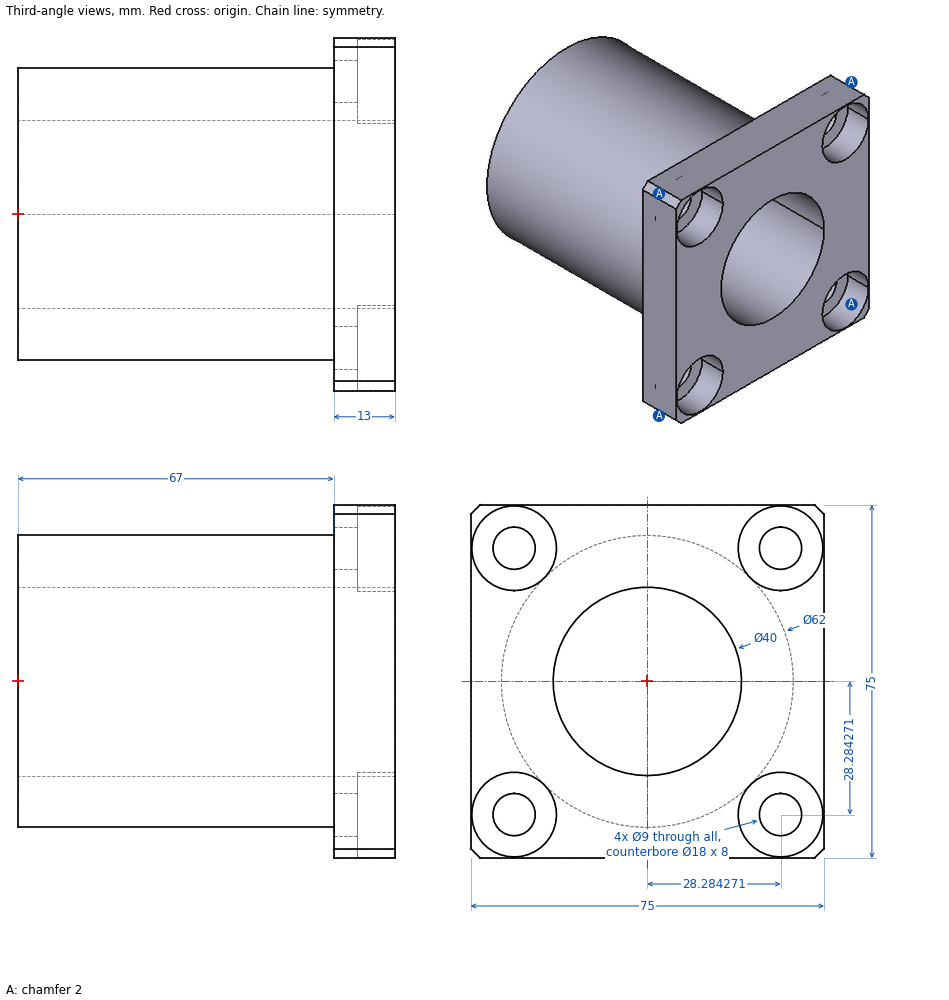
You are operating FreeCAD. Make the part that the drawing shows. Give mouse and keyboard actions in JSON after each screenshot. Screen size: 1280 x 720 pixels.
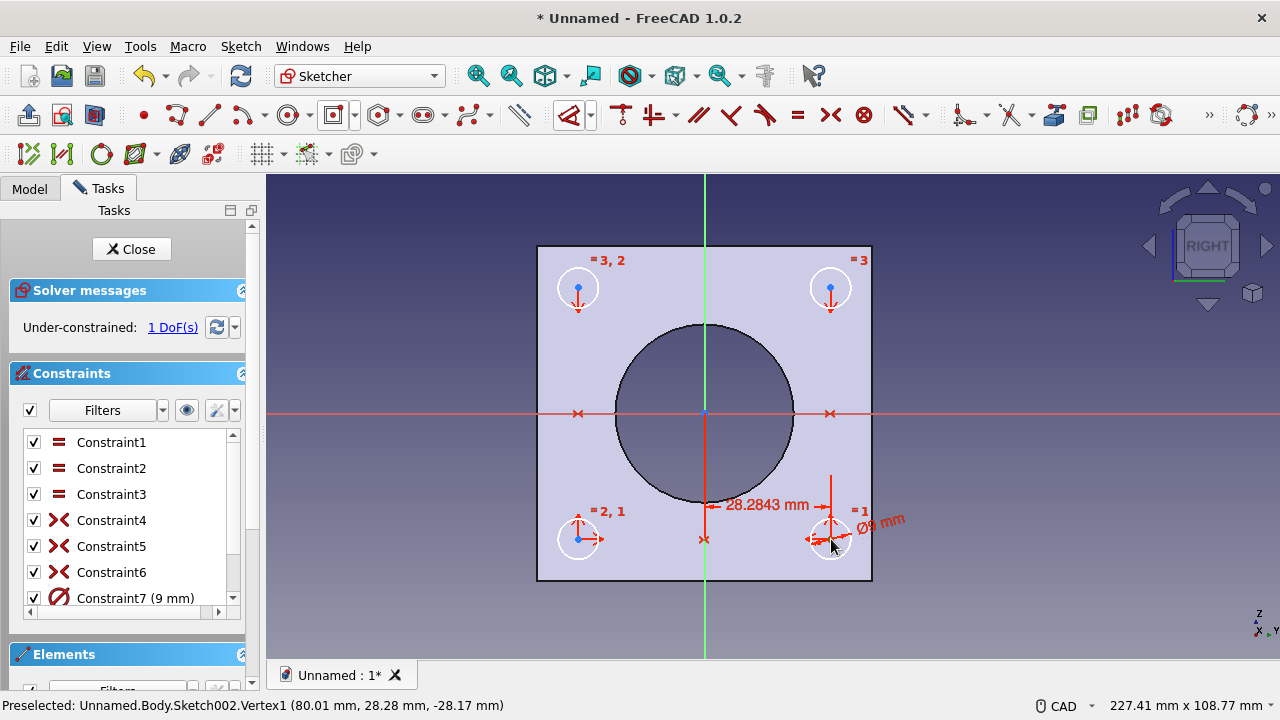
{"action": "key", "text": "i"}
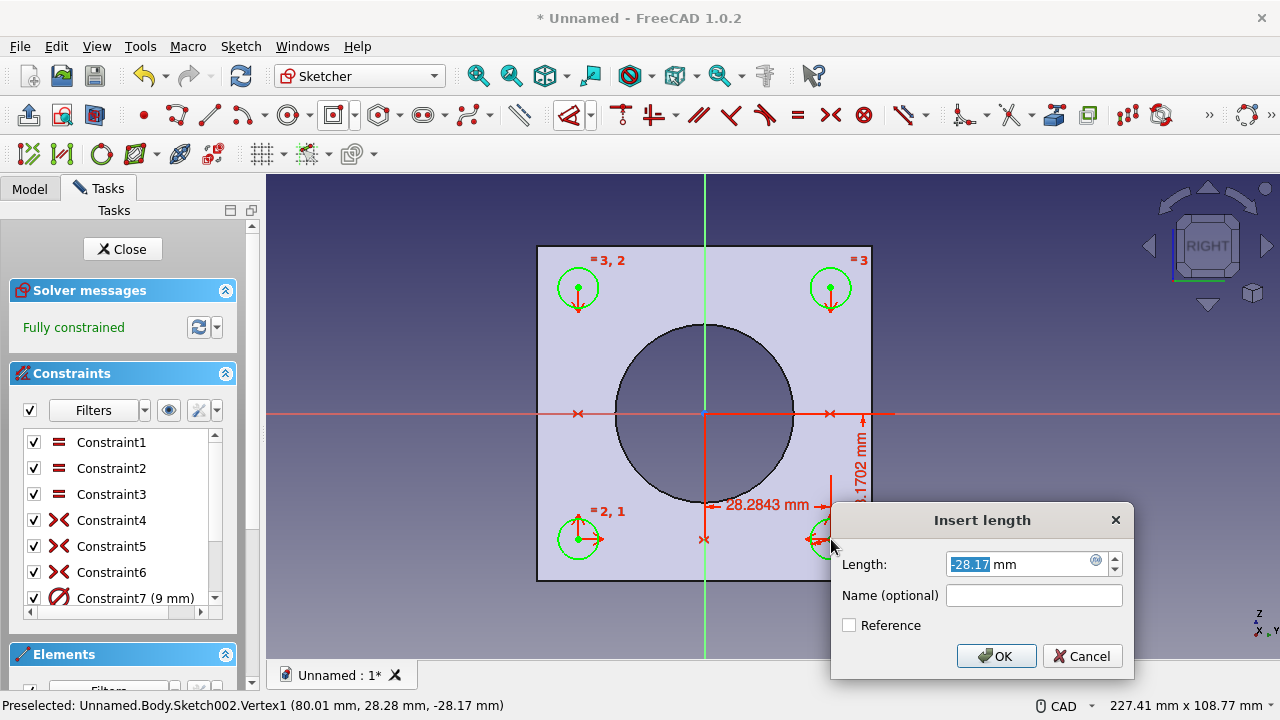
{"action": "type", "text": "-28.284271"}
{"action": "key", "text": "Return"}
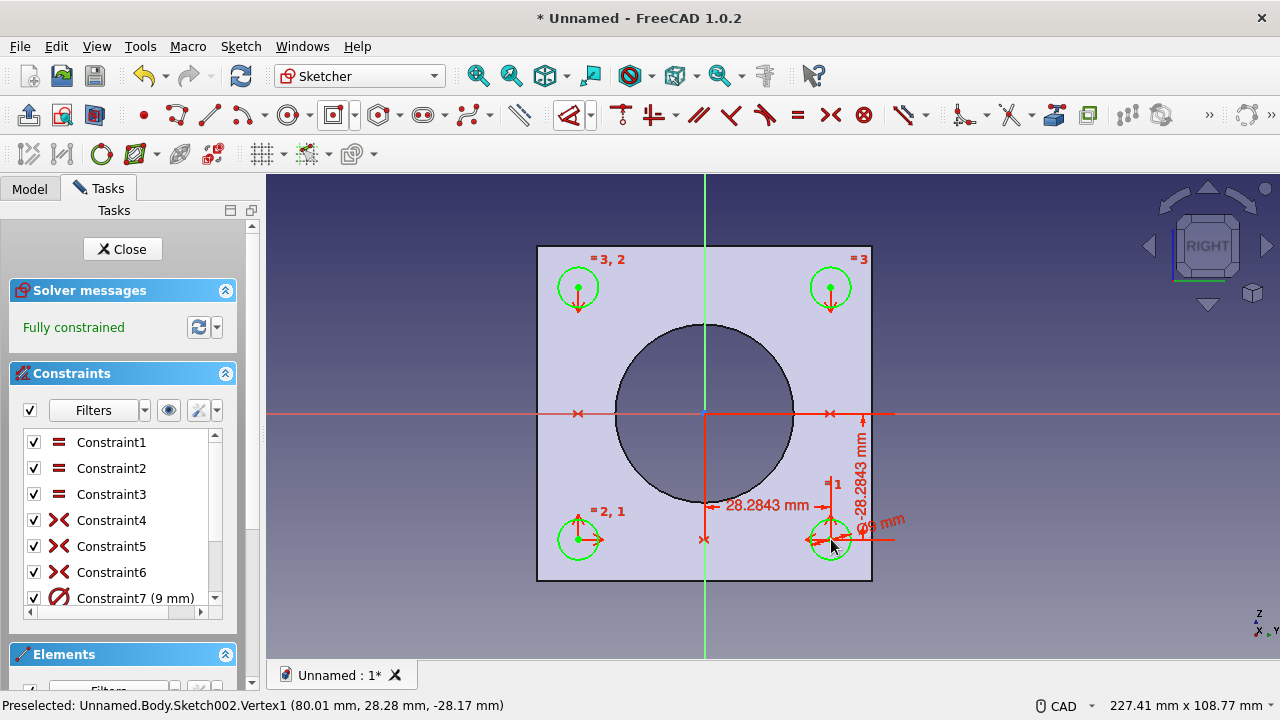
{"action": "left_click", "coordinate": [123, 249]}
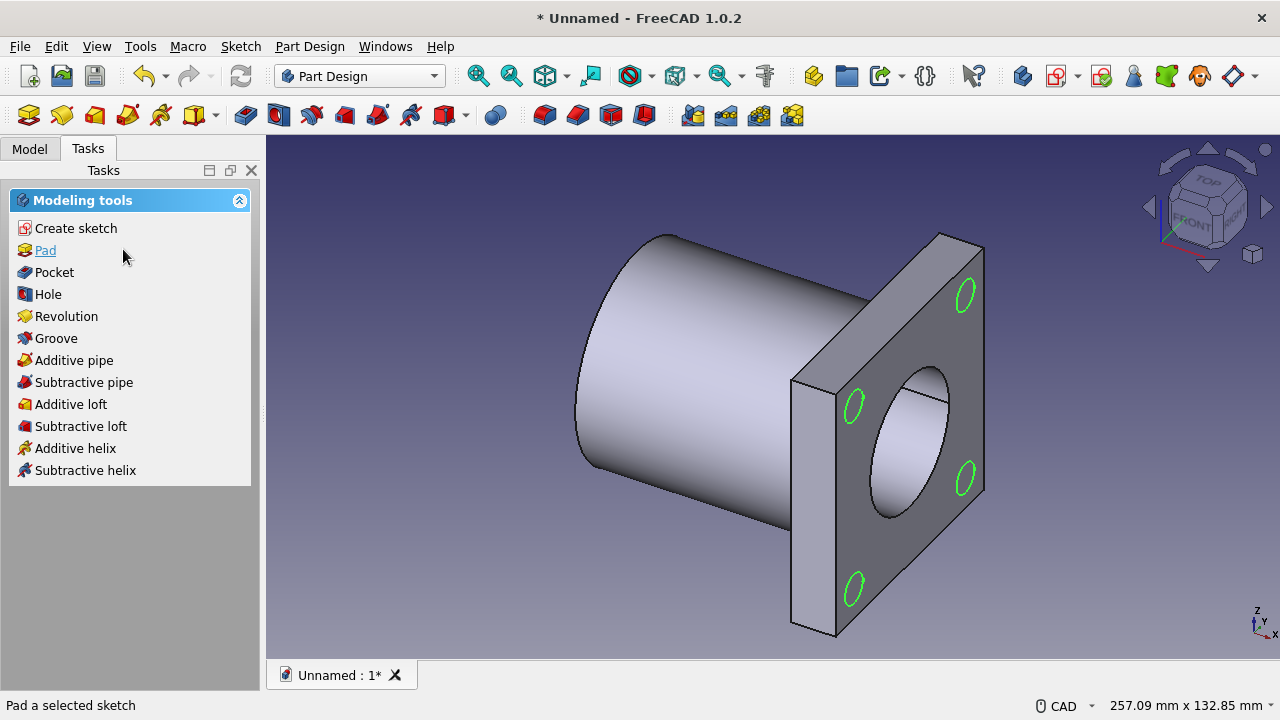
{"action": "left_click", "coordinate": [279, 116]}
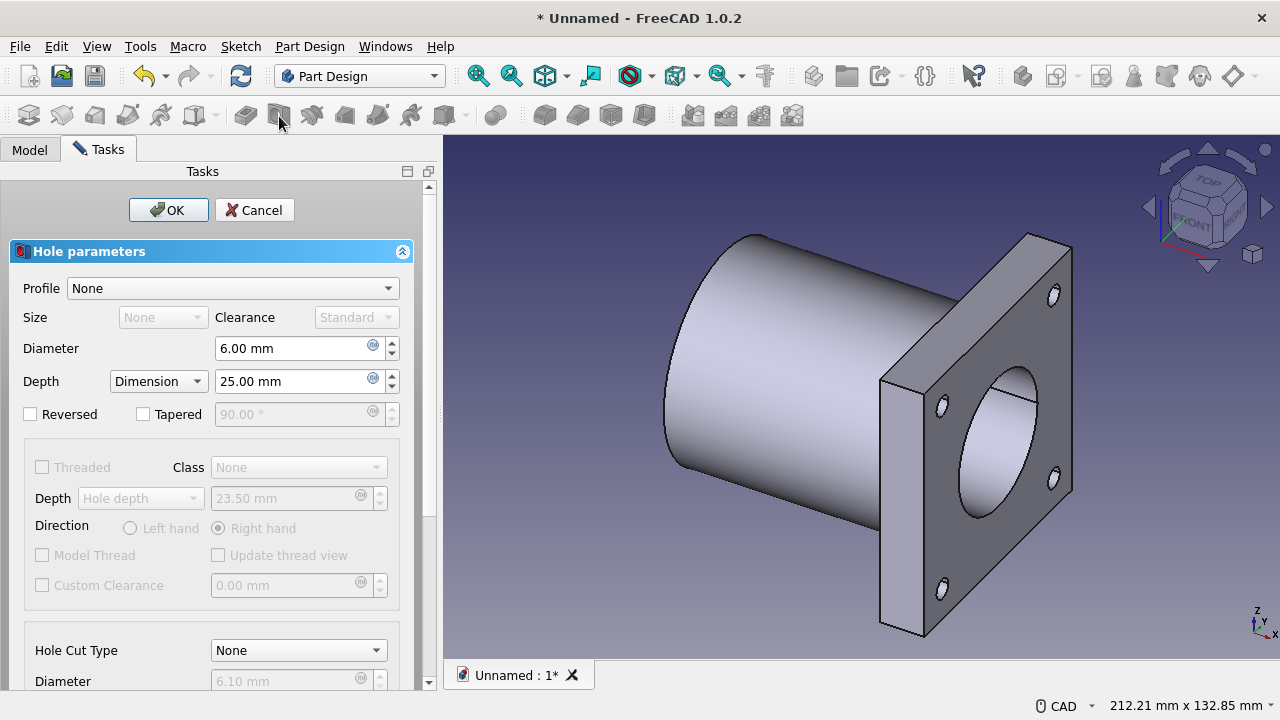
{"action": "triple_click", "coordinate": [300, 348]}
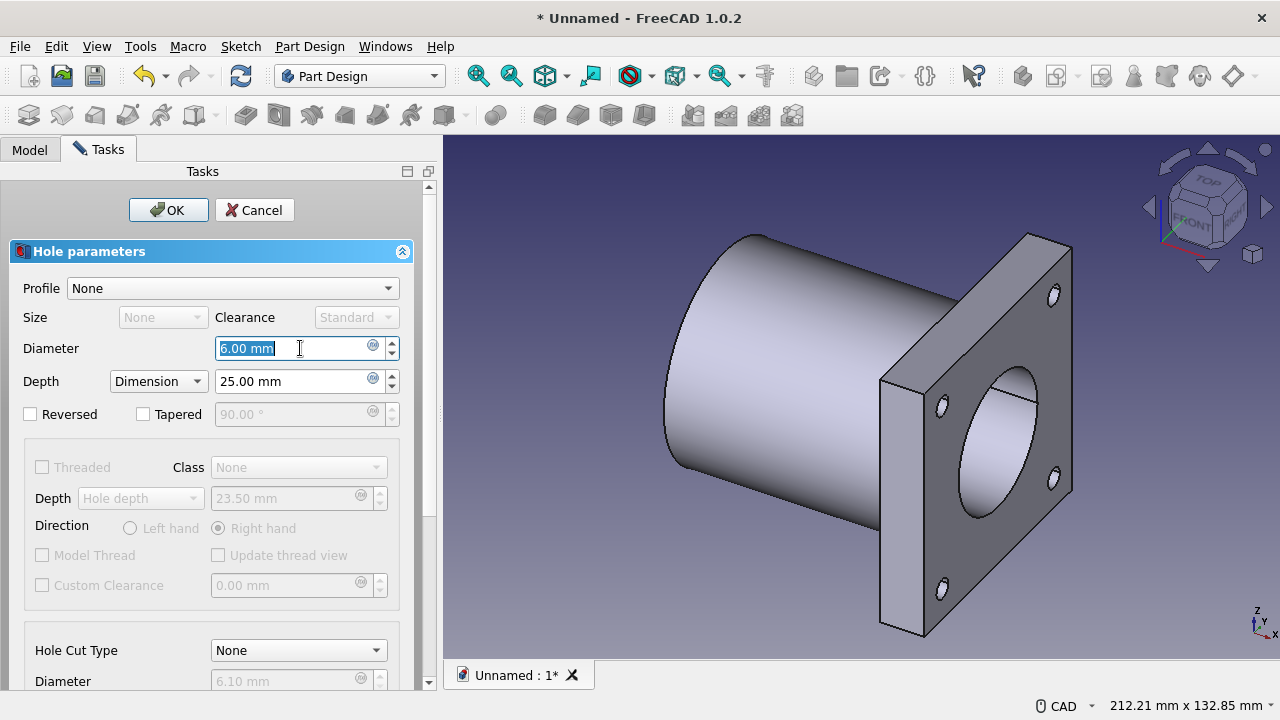
{"action": "type", "text": "9"}
{"action": "key", "text": "Tab"}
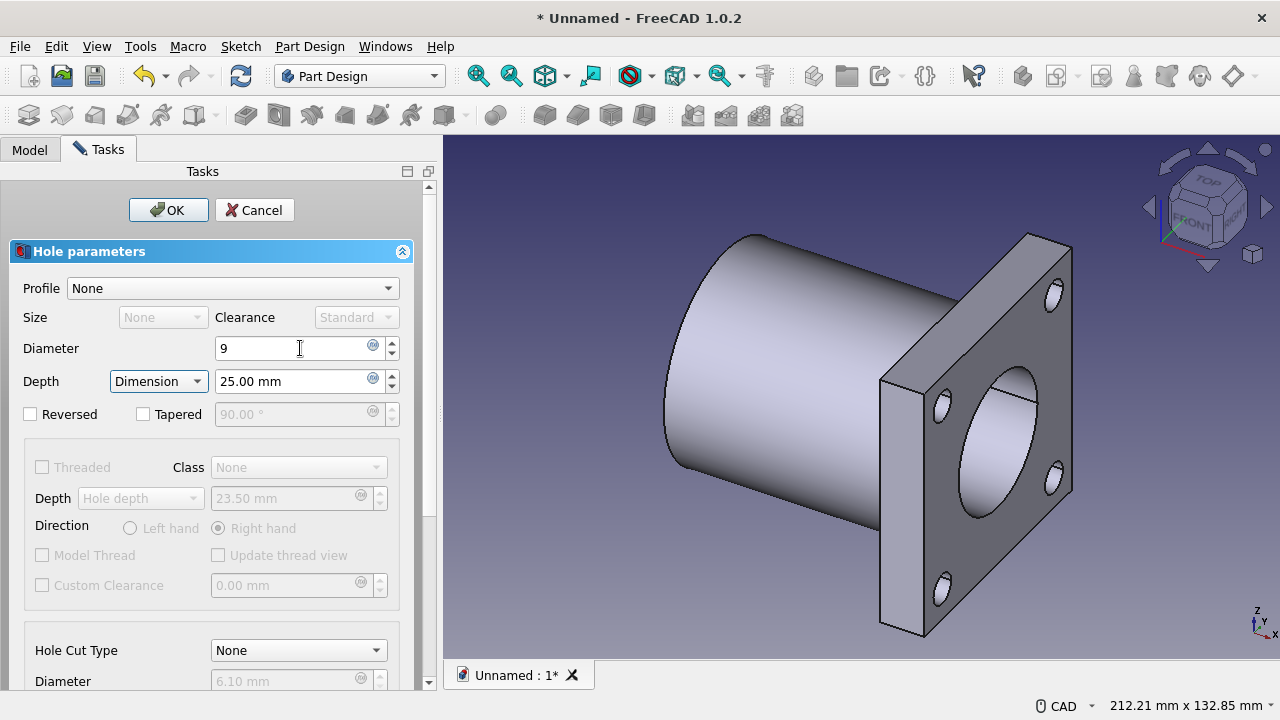
{"action": "left_click", "coordinate": [160, 382]}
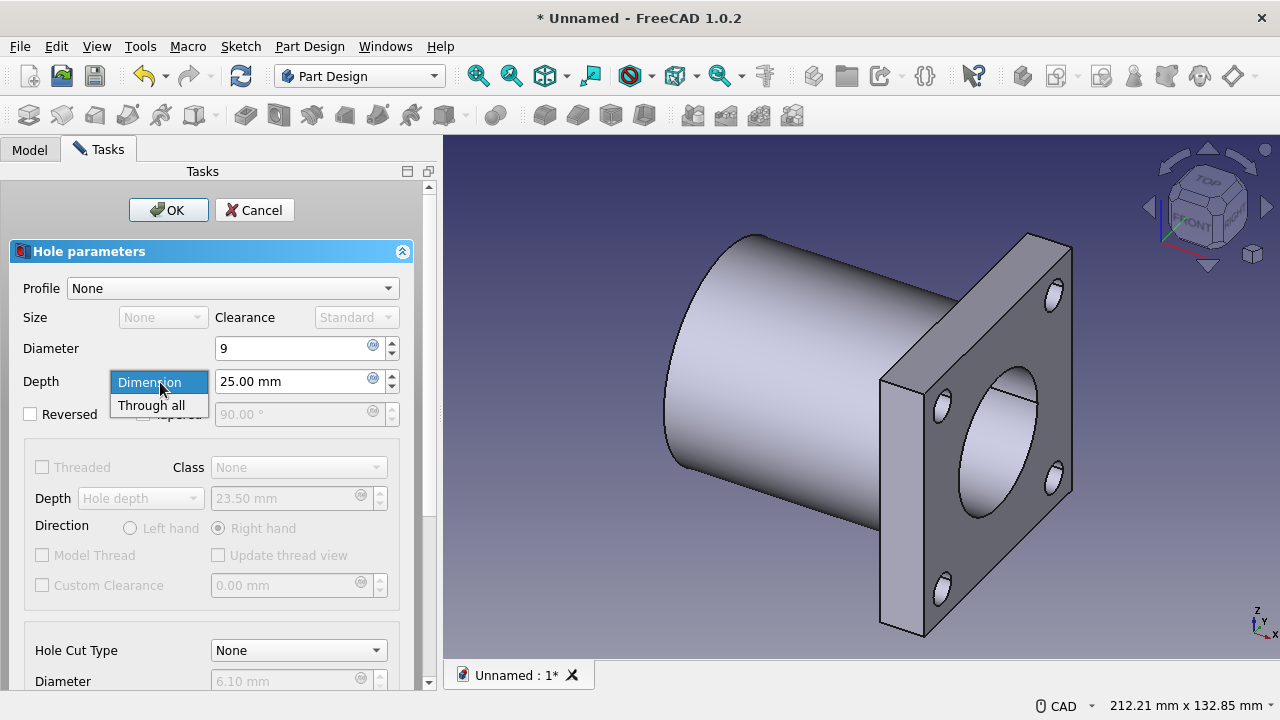
{"action": "left_click", "coordinate": [158, 406]}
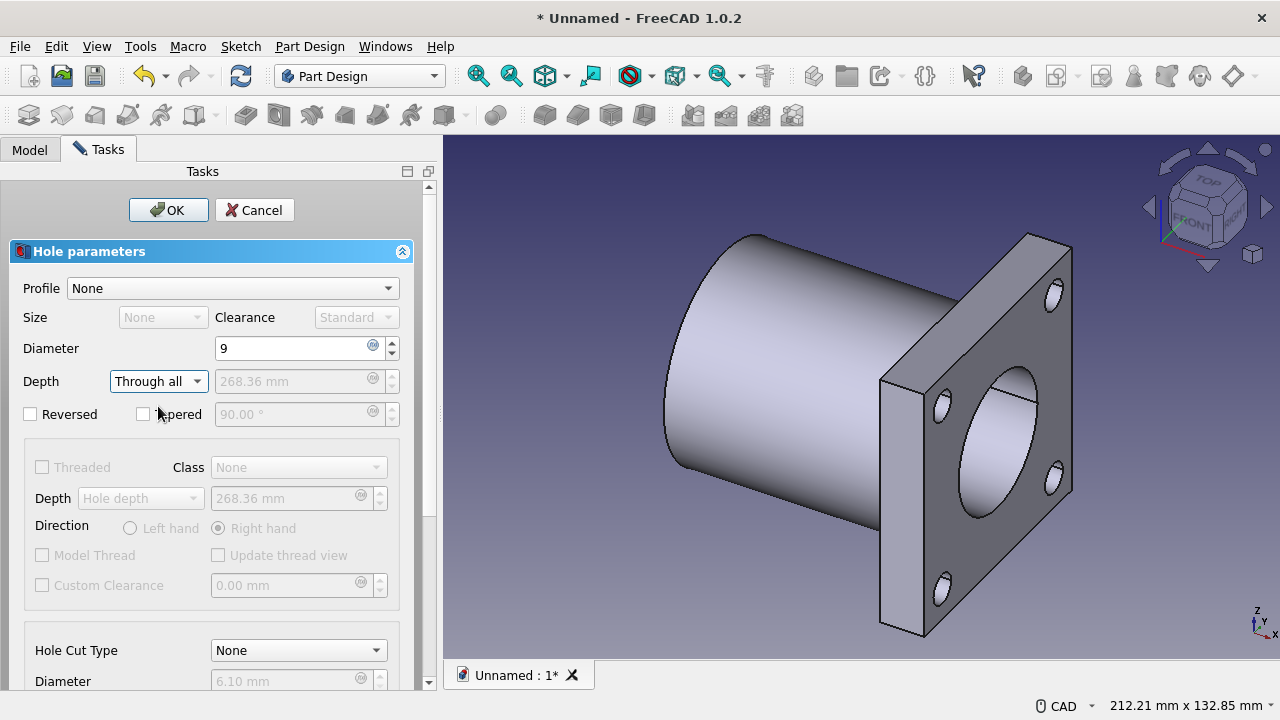
{"action": "left_click", "coordinate": [300, 650]}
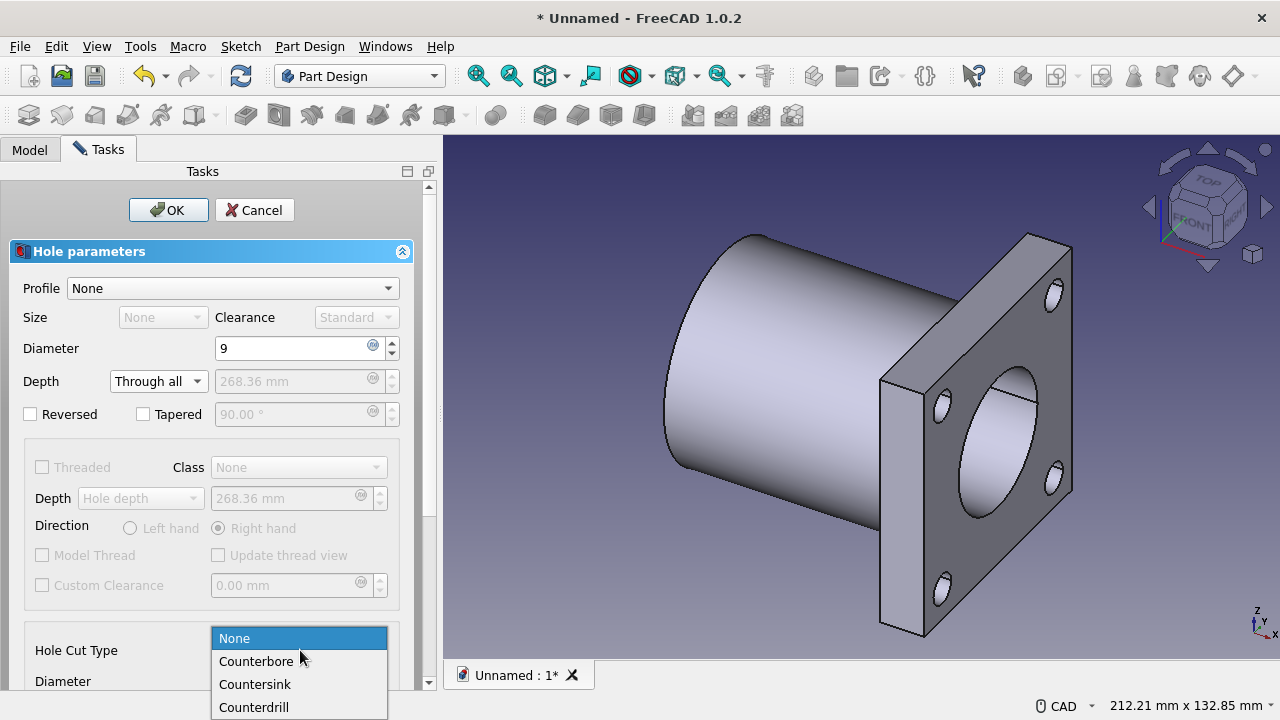
{"action": "left_click", "coordinate": [298, 662]}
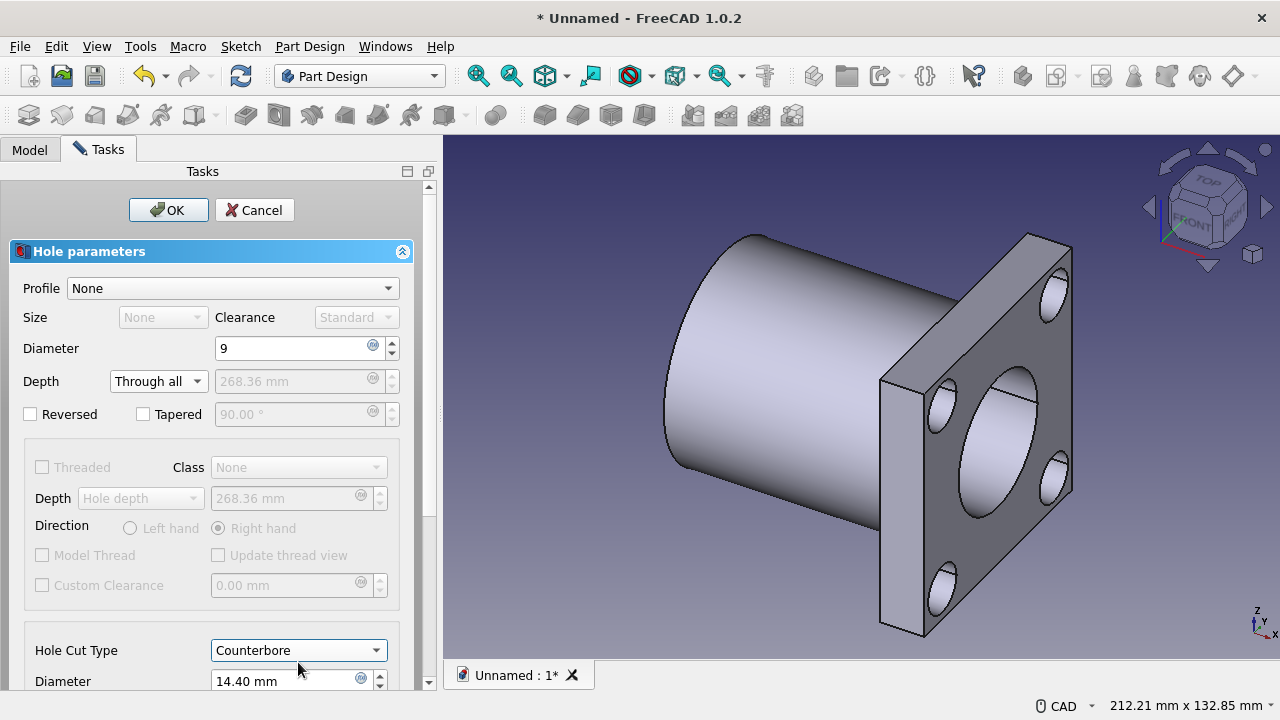
{"action": "scroll", "coordinate": [429, 436], "scroll_direction": "down", "scroll_amount": 2}